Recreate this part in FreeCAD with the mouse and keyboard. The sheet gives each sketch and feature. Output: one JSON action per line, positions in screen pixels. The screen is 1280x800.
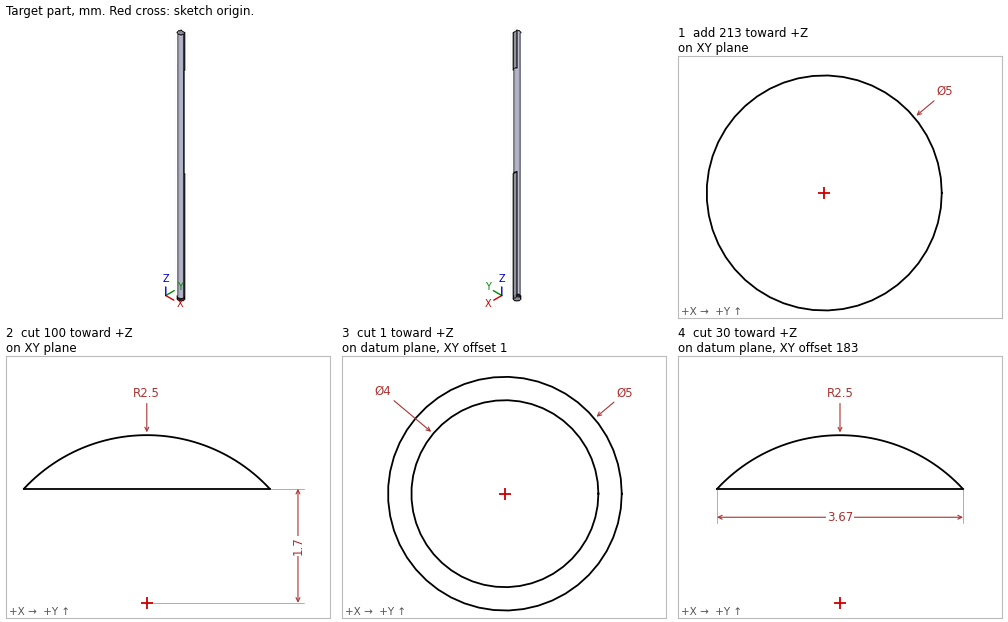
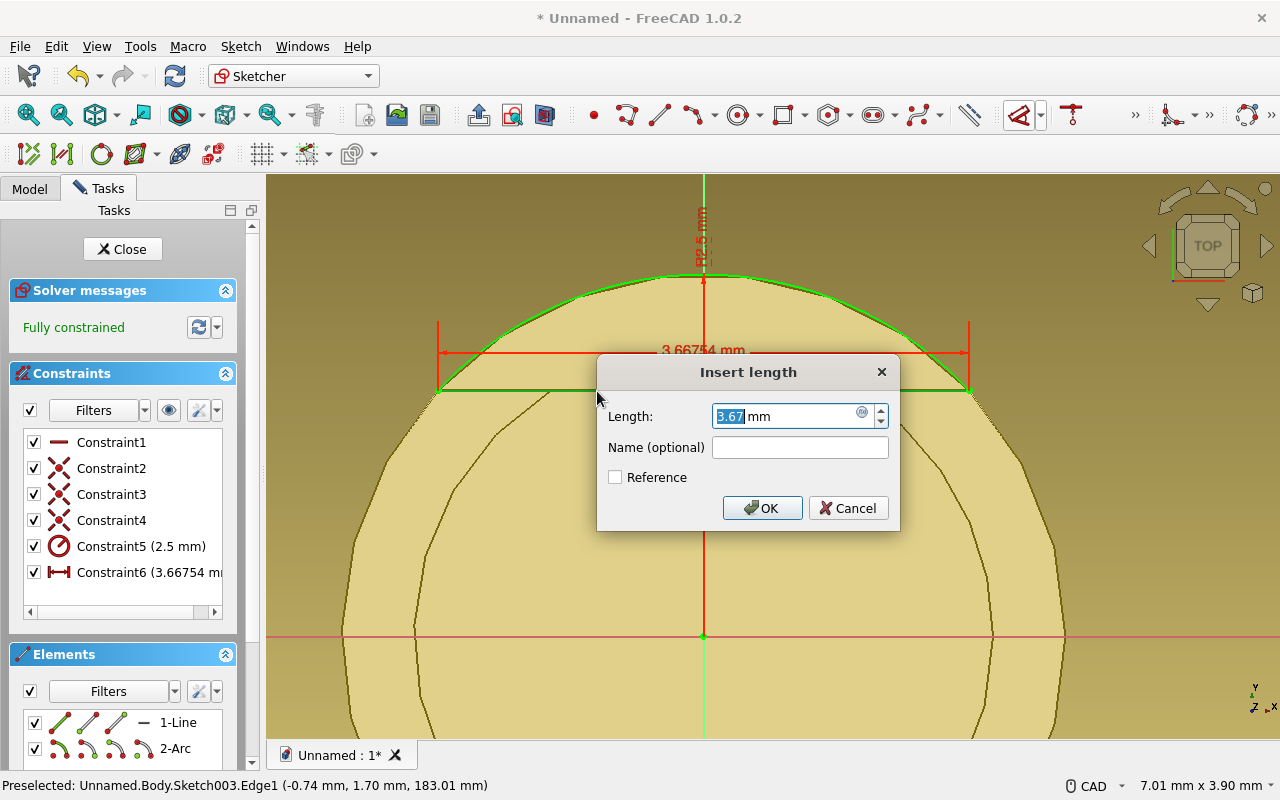
{"action": "type", "text": "3.67"}
{"action": "key", "text": "Return"}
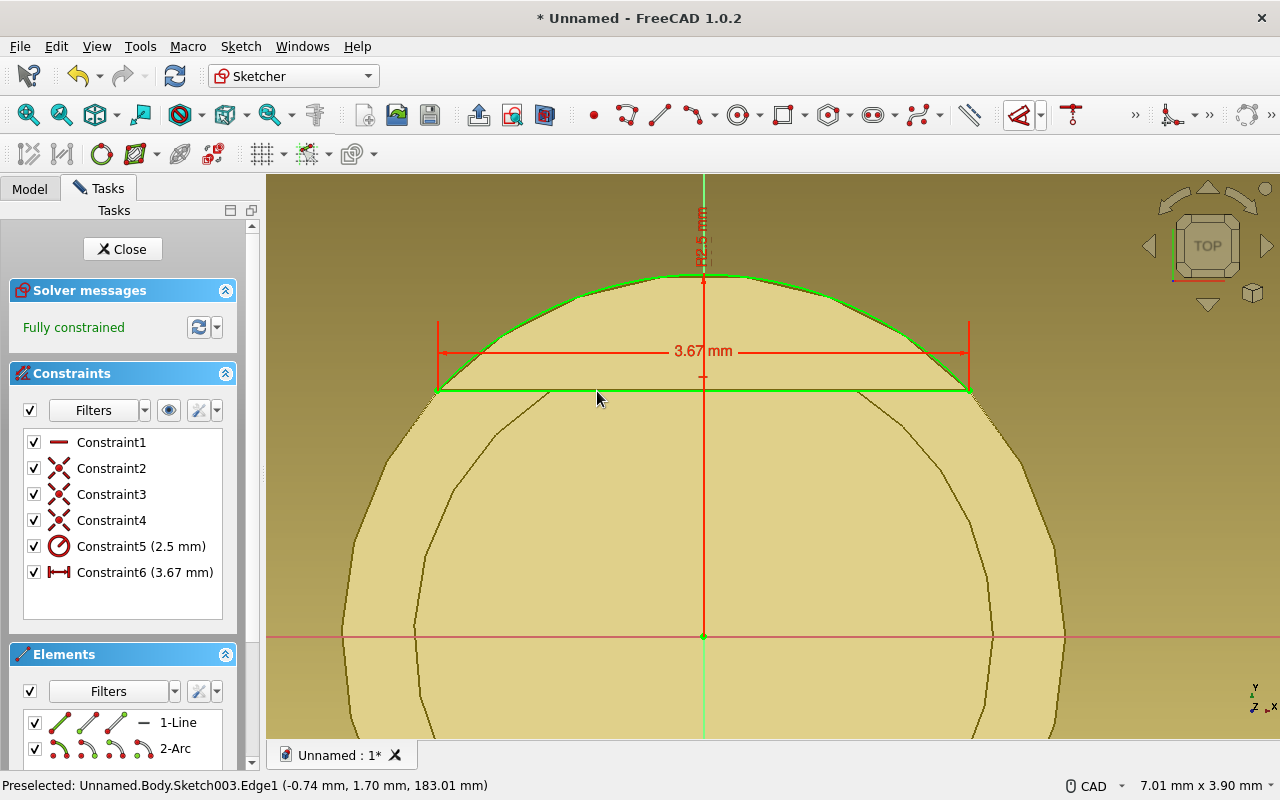
{"action": "left_click", "coordinate": [123, 249]}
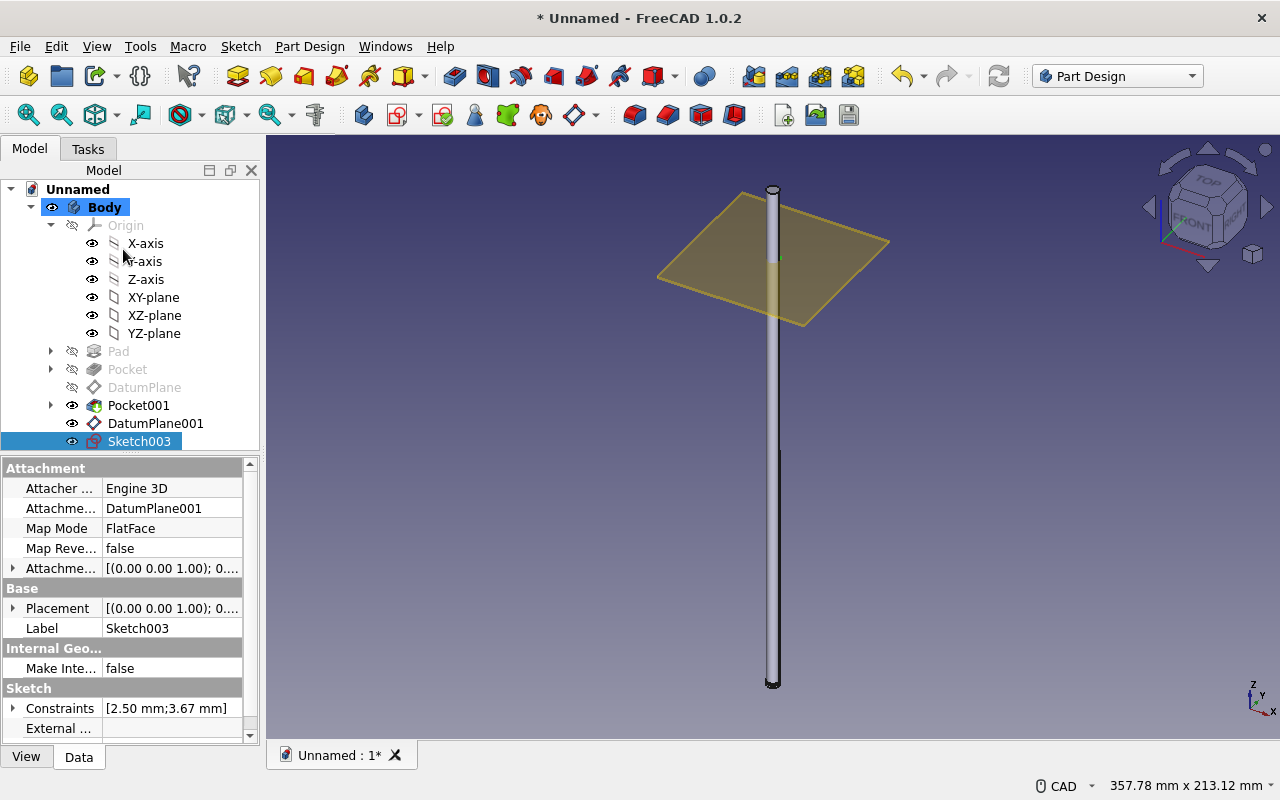
{"action": "left_click", "coordinate": [455, 76]}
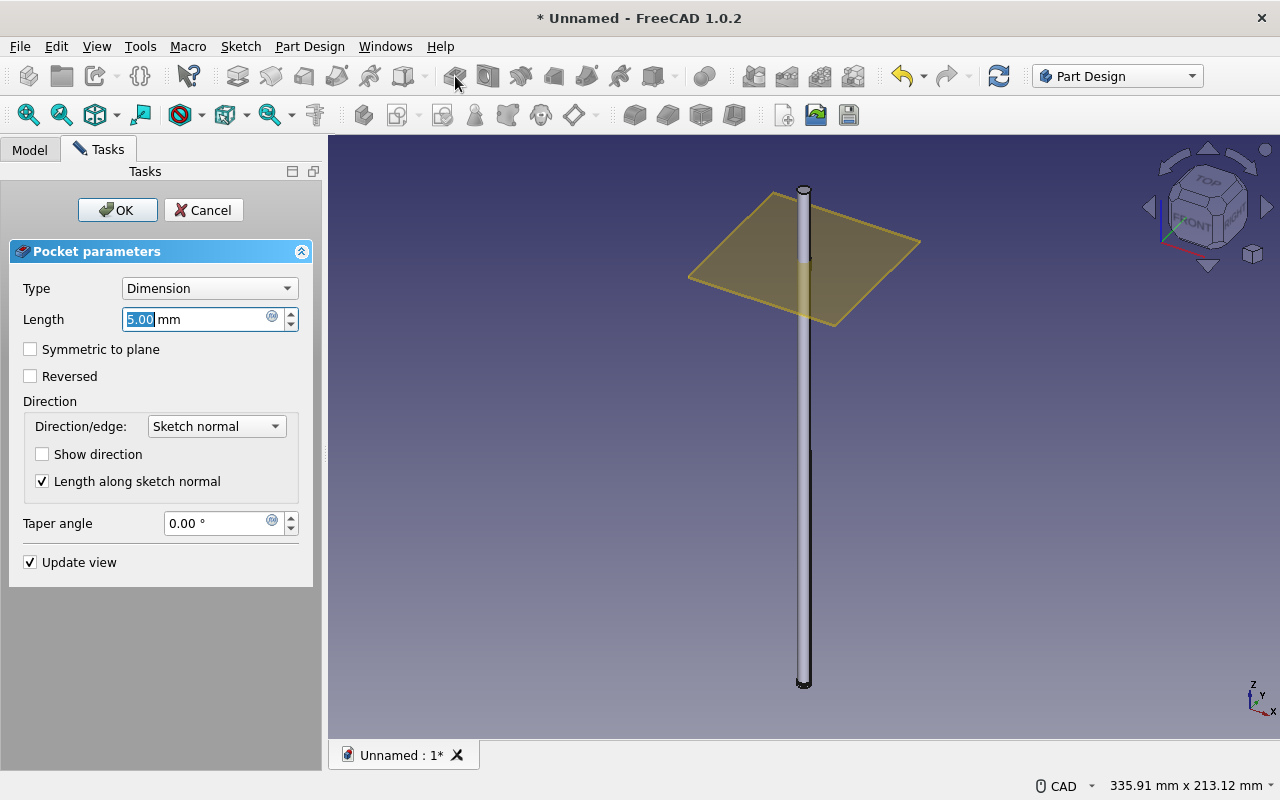
{"action": "type", "text": "30"}
{"action": "key", "text": "Tab"}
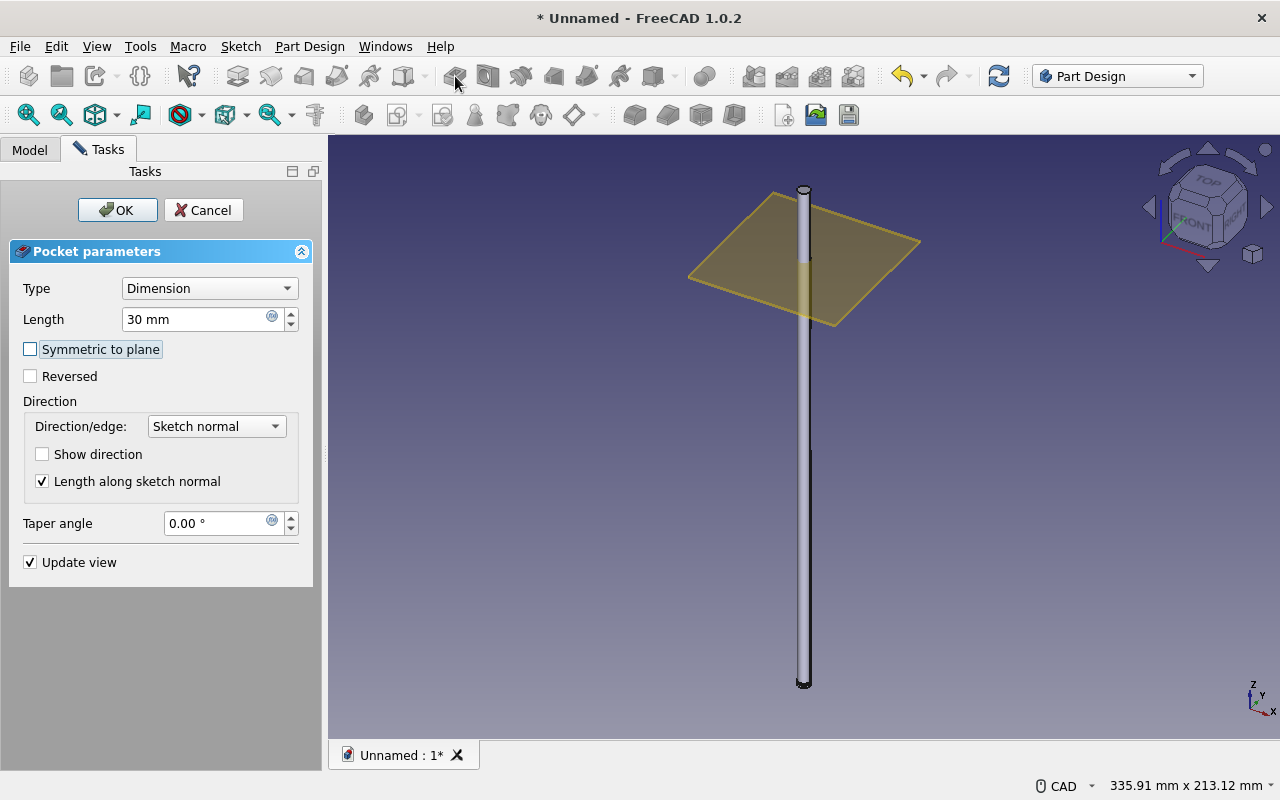
{"action": "left_click", "coordinate": [31, 376]}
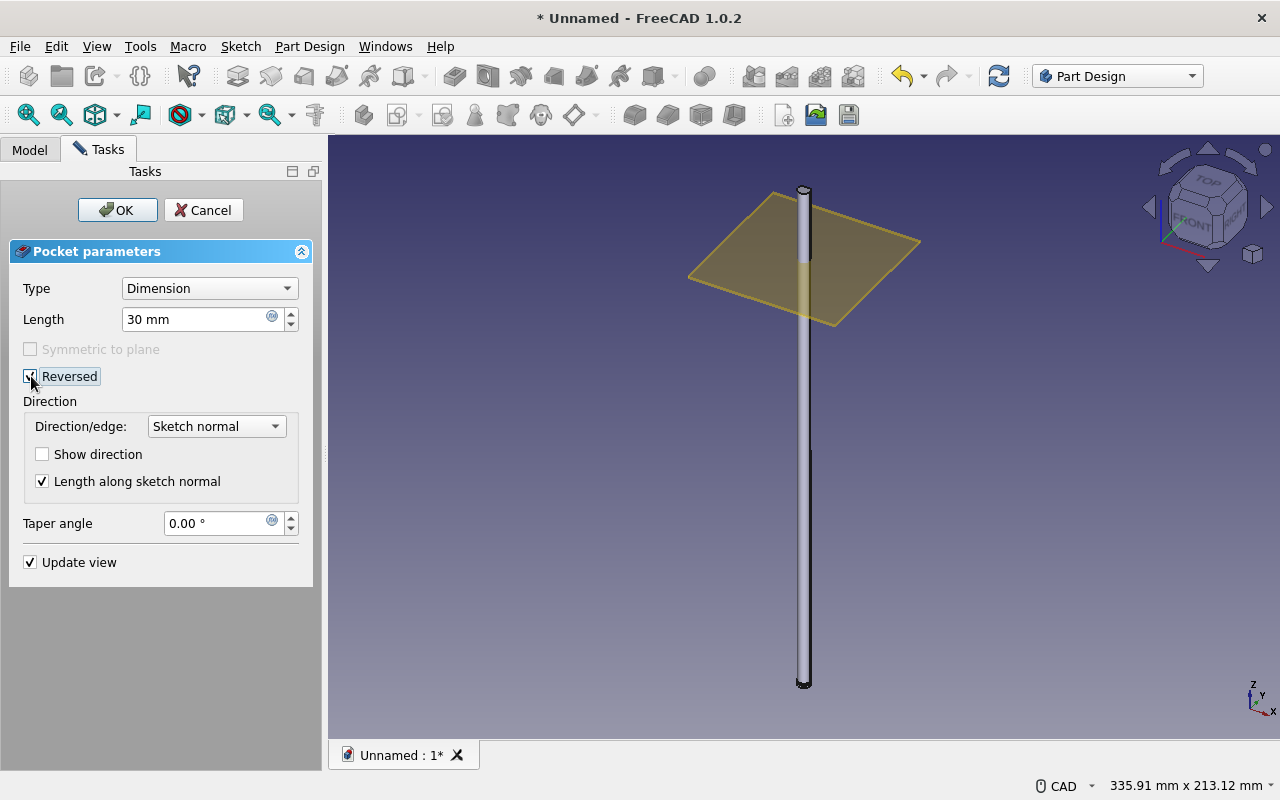
{"action": "left_click", "coordinate": [118, 210]}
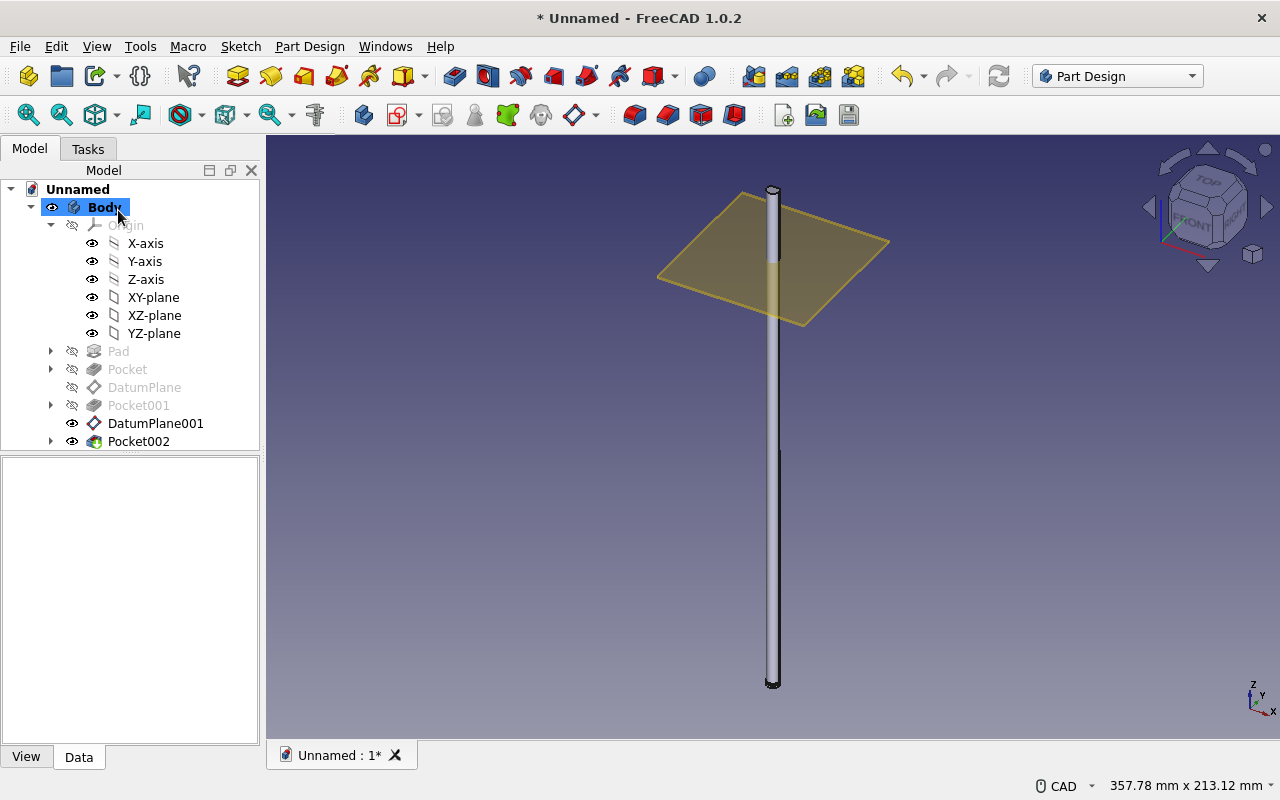
{"action": "left_click", "coordinate": [117, 423]}
{"action": "key", "text": "space"}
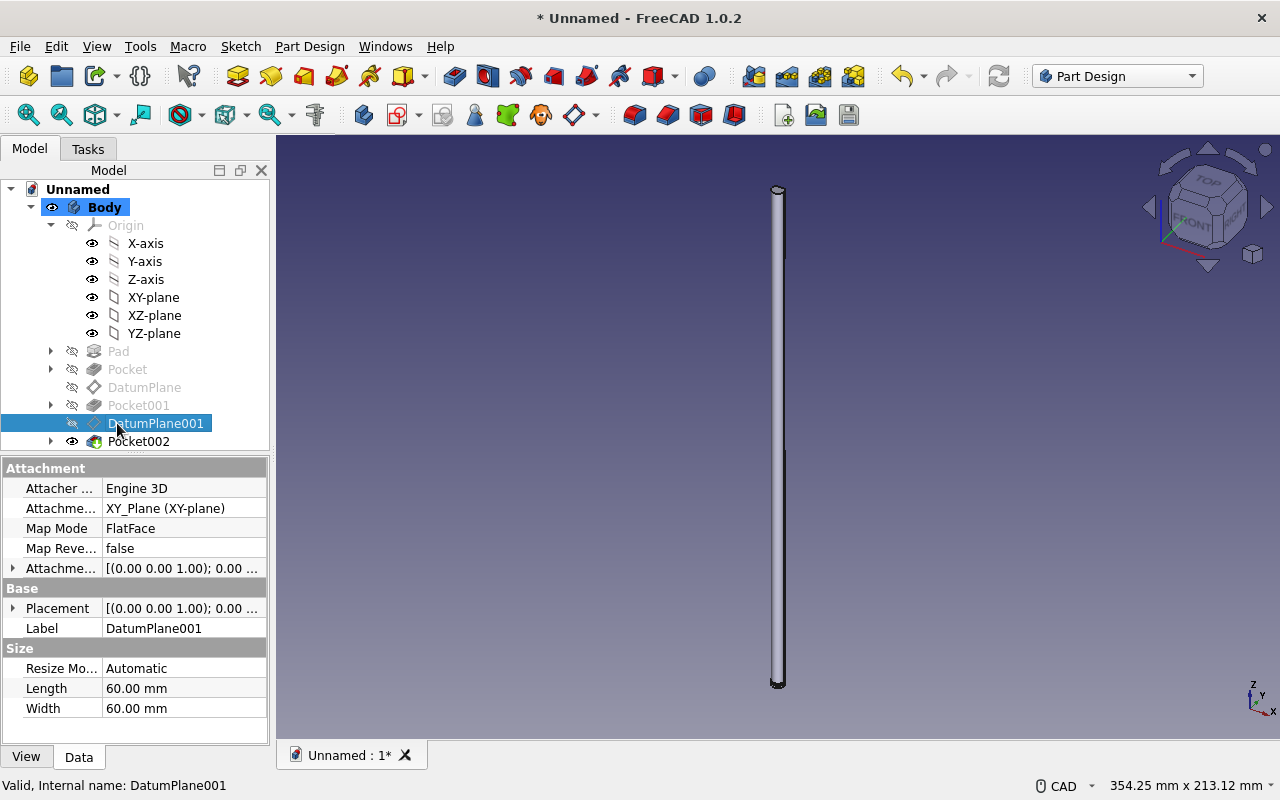
{"action": "key", "text": "0"}